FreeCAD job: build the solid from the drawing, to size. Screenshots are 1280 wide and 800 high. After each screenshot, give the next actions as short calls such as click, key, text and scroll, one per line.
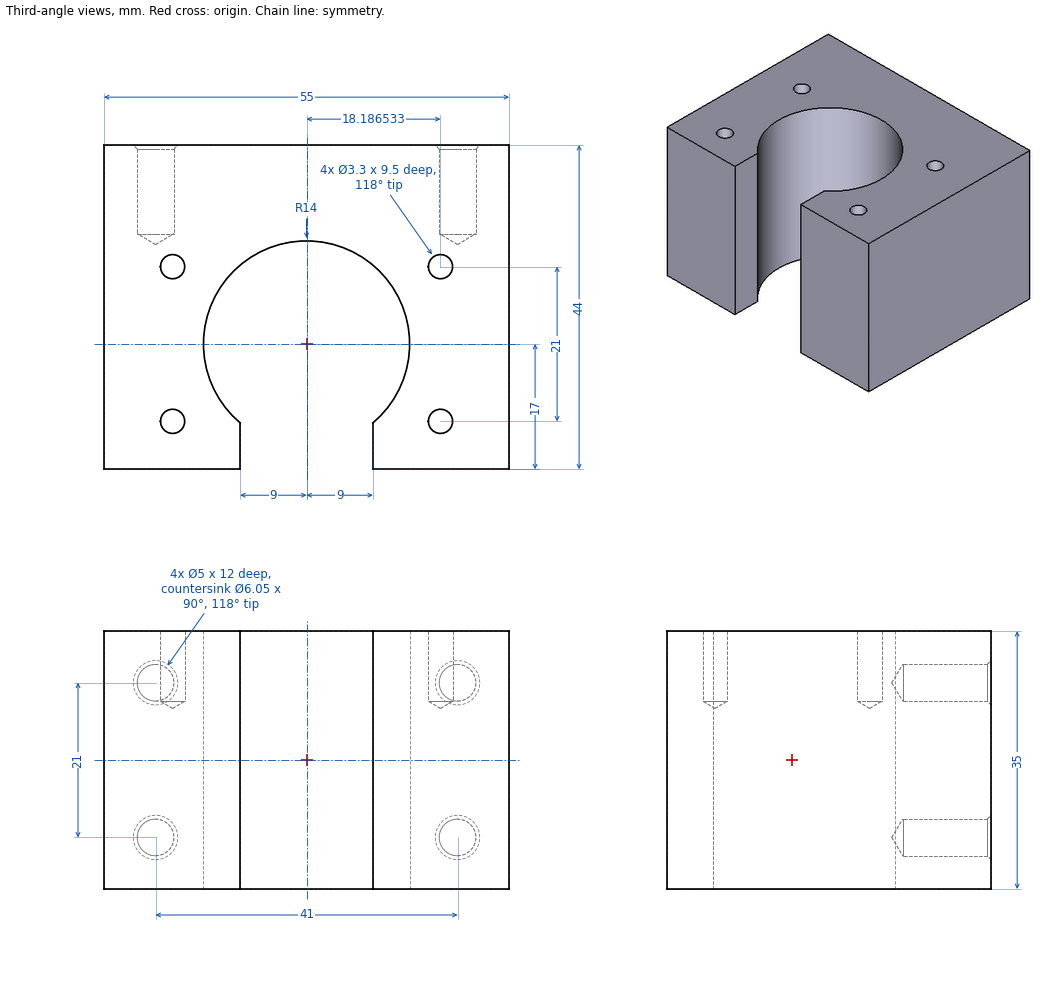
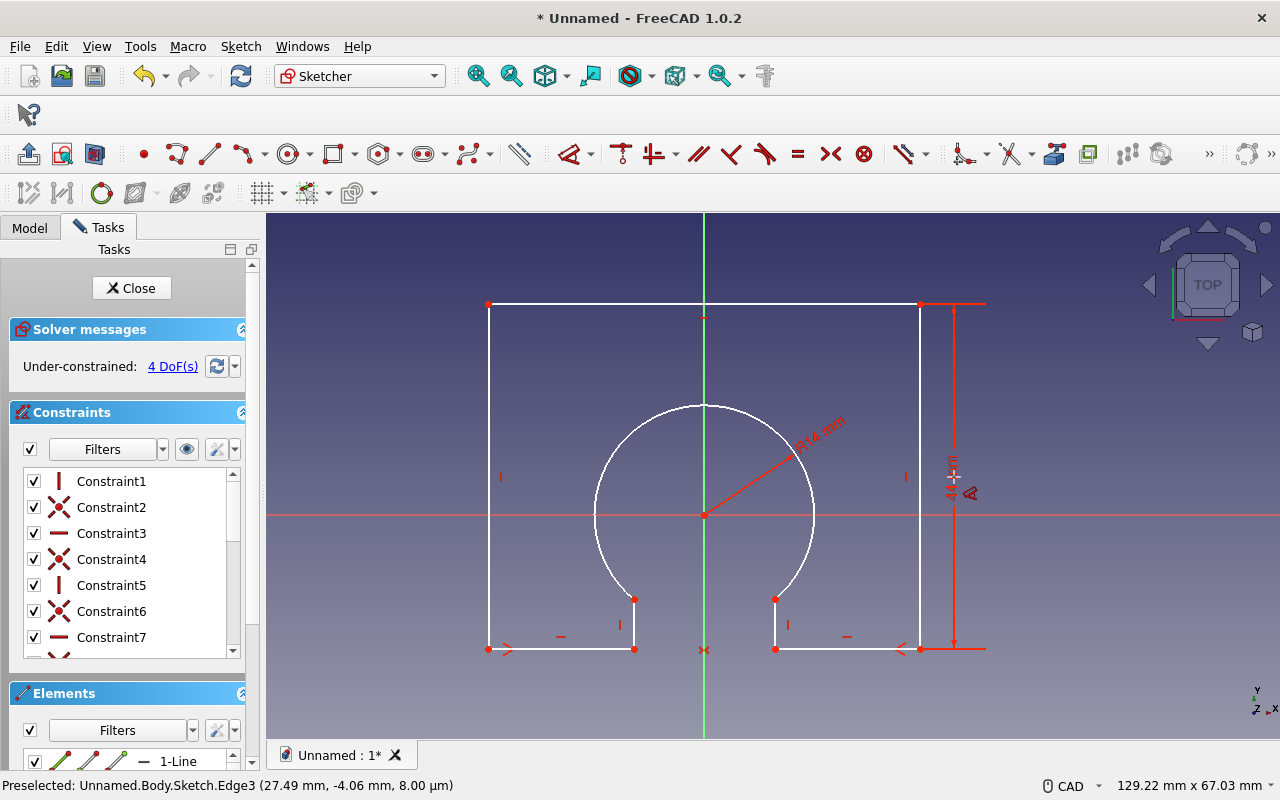
click(791, 304)
click(605, 270)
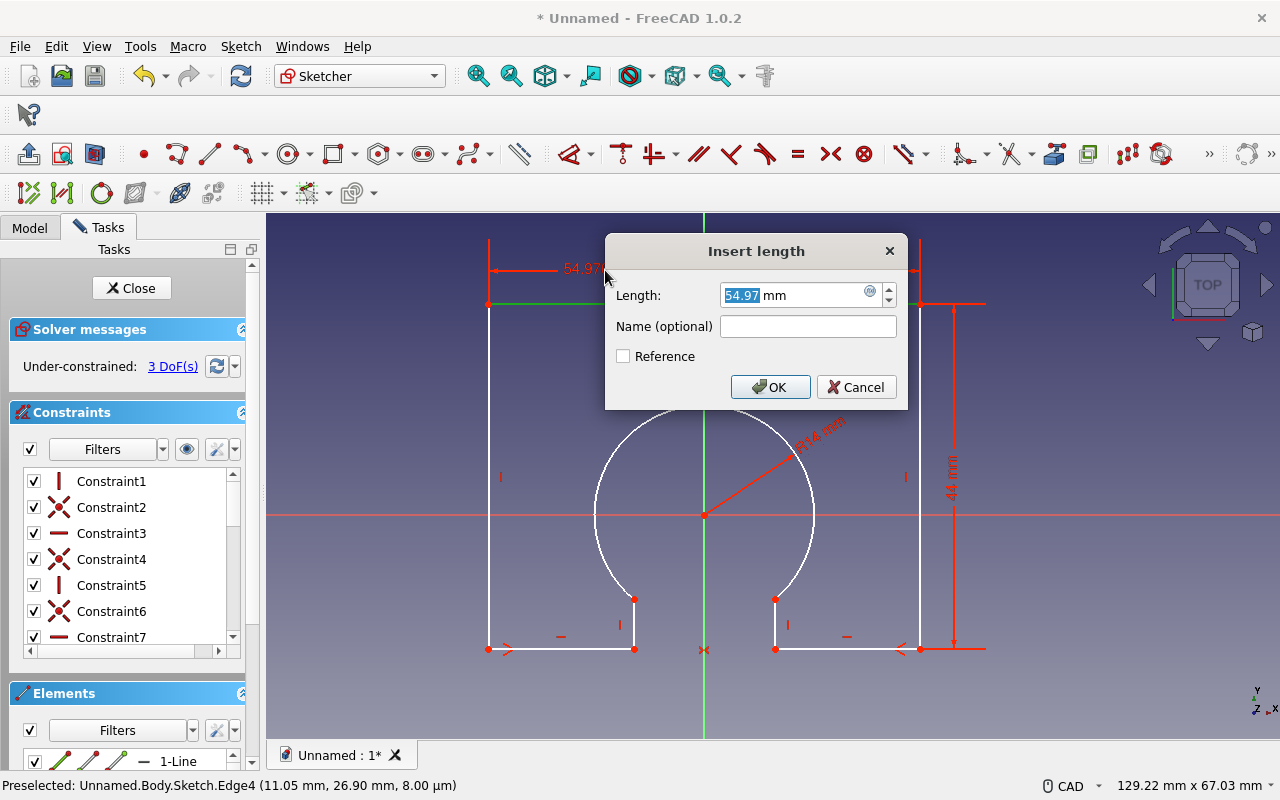
text(55)
key(Return)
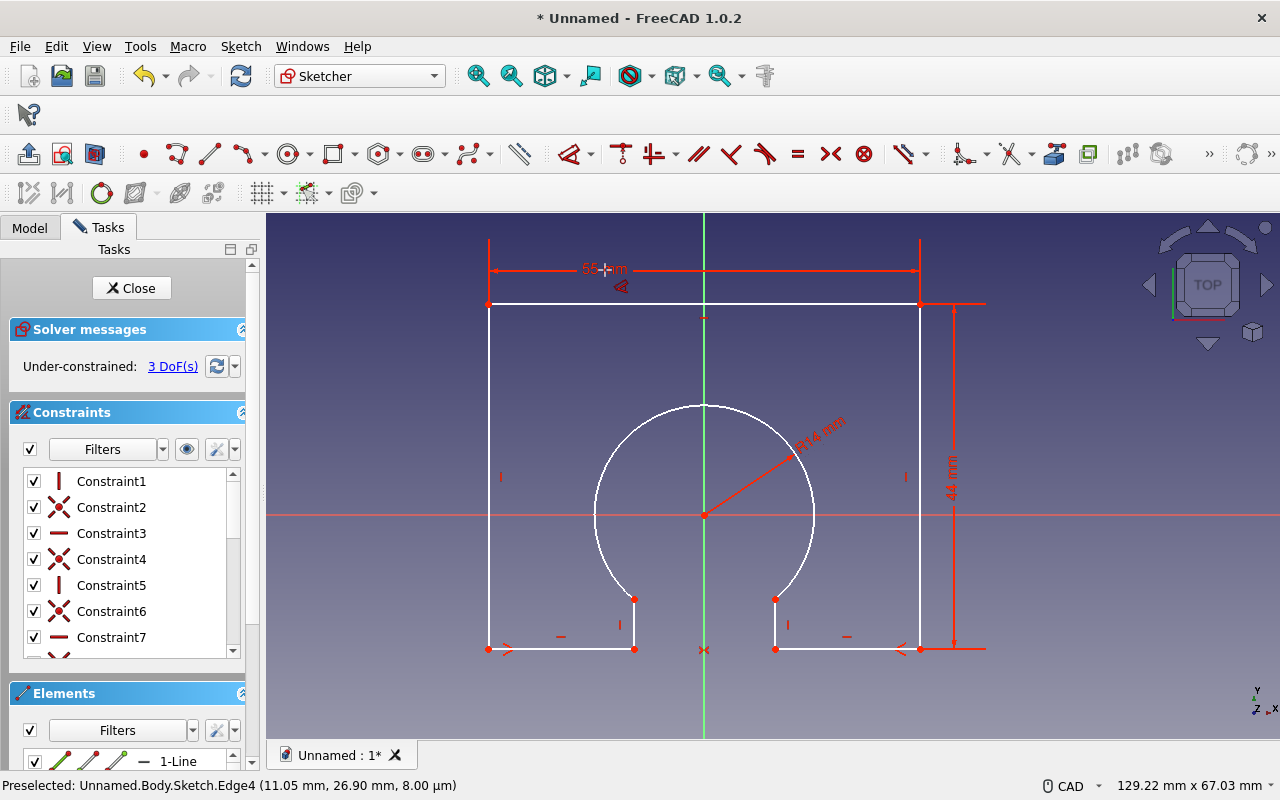
click(775, 599)
click(740, 633)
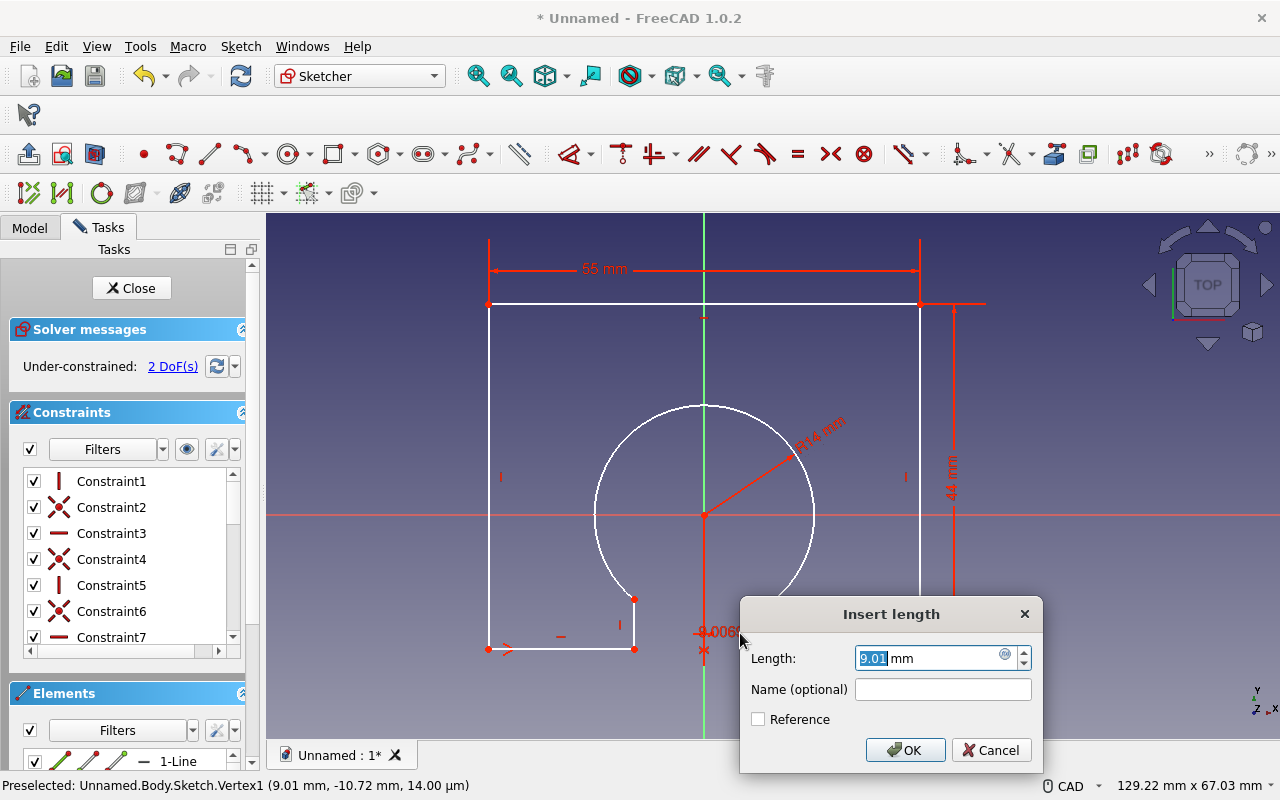
text(9)
key(Return)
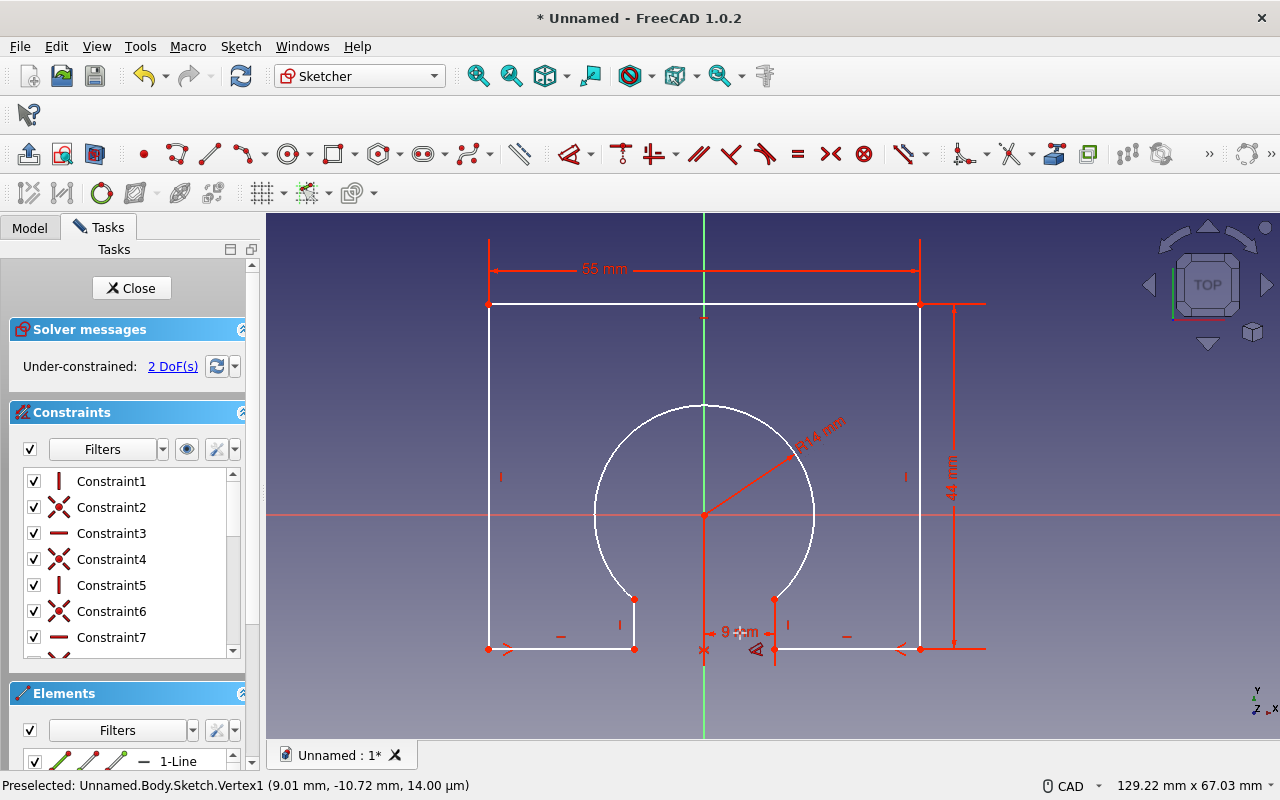
click(634, 649)
click(669, 683)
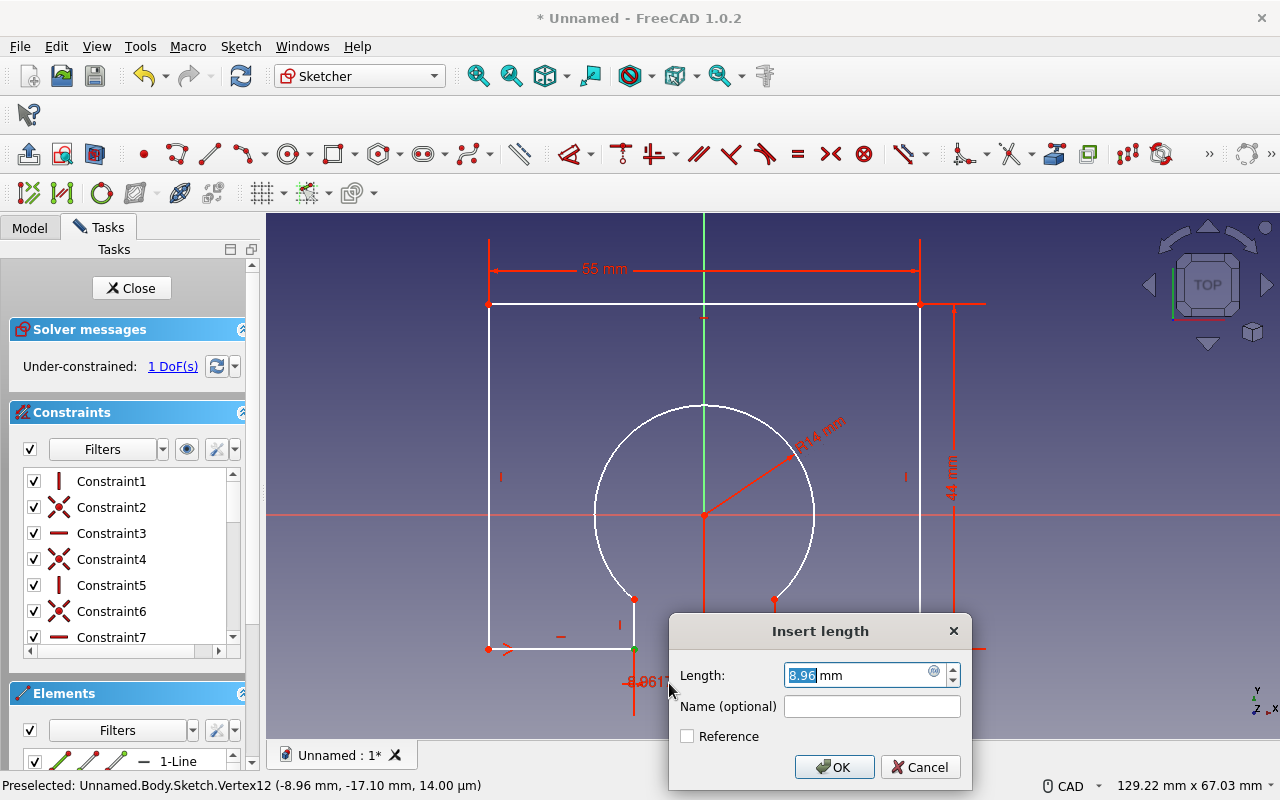
text(9)
key(Return)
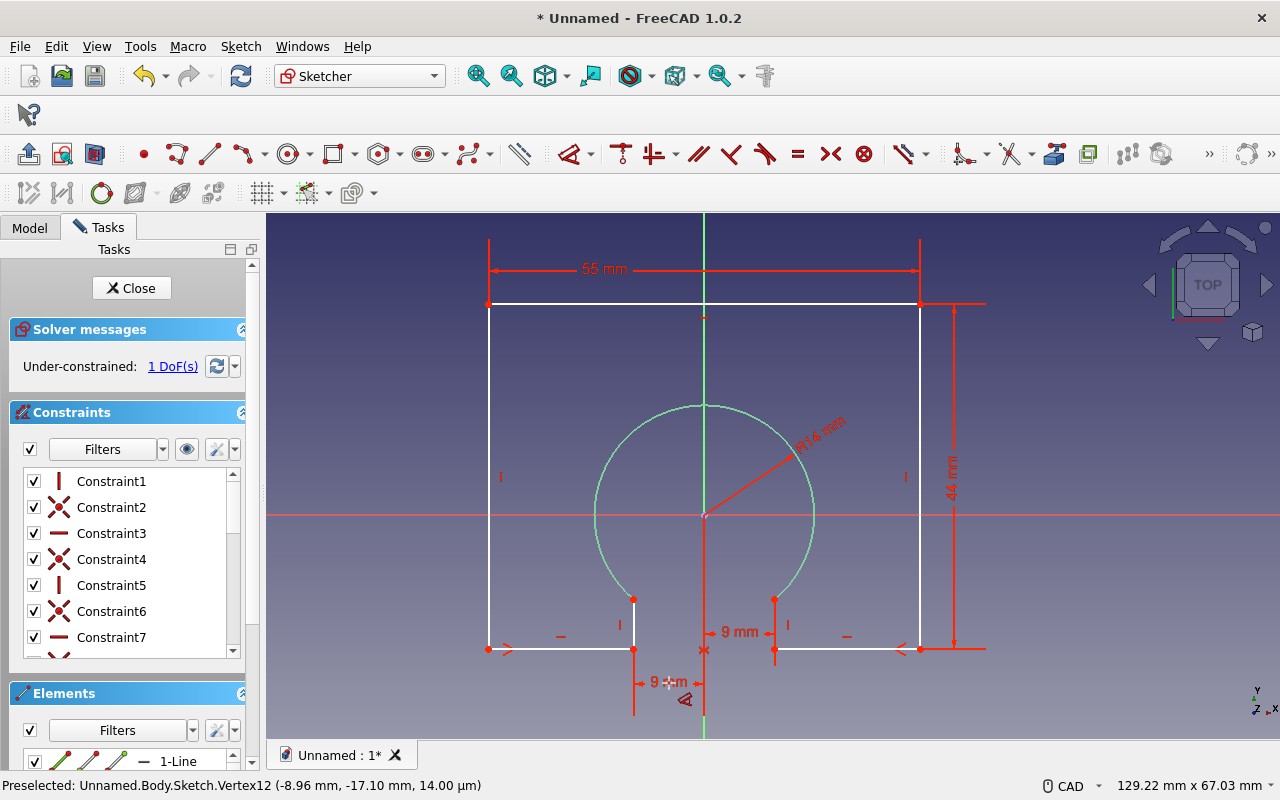
click(775, 649)
click(809, 582)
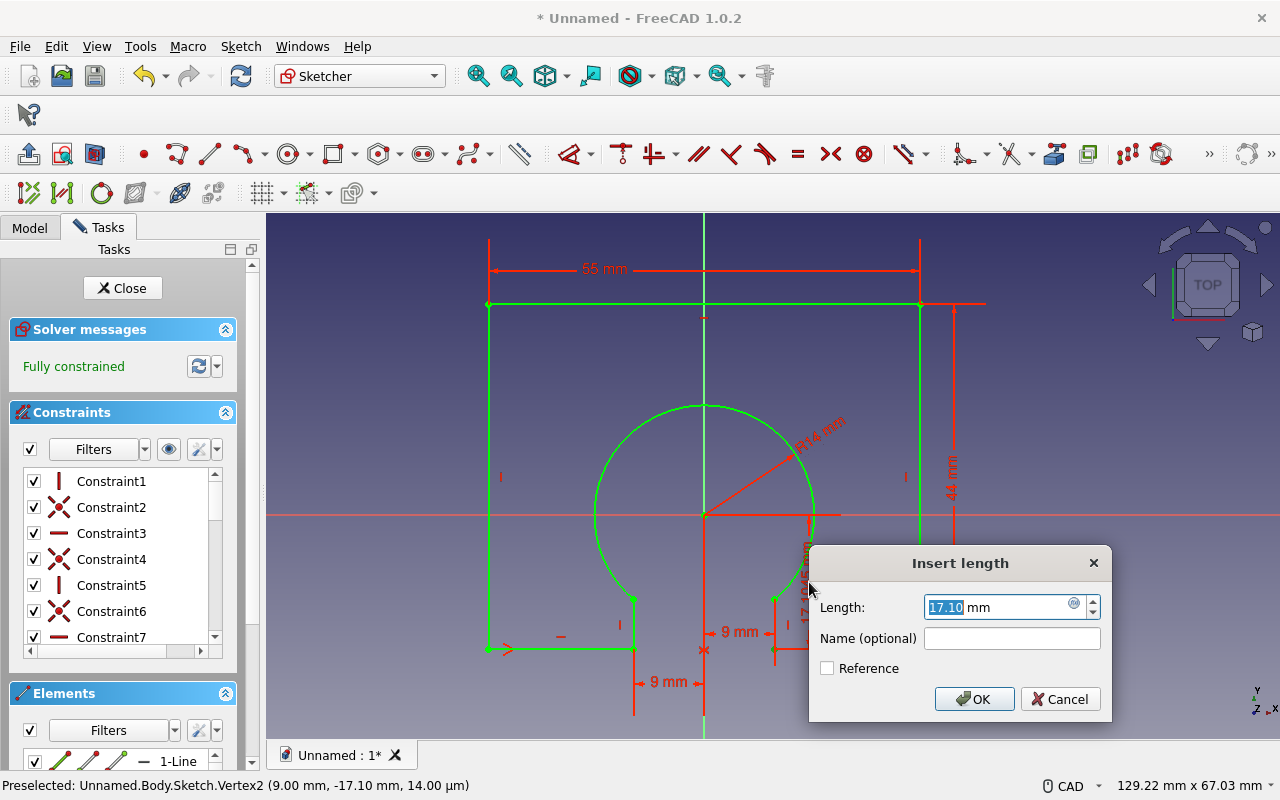
text(17)
key(Return)
key(Escape)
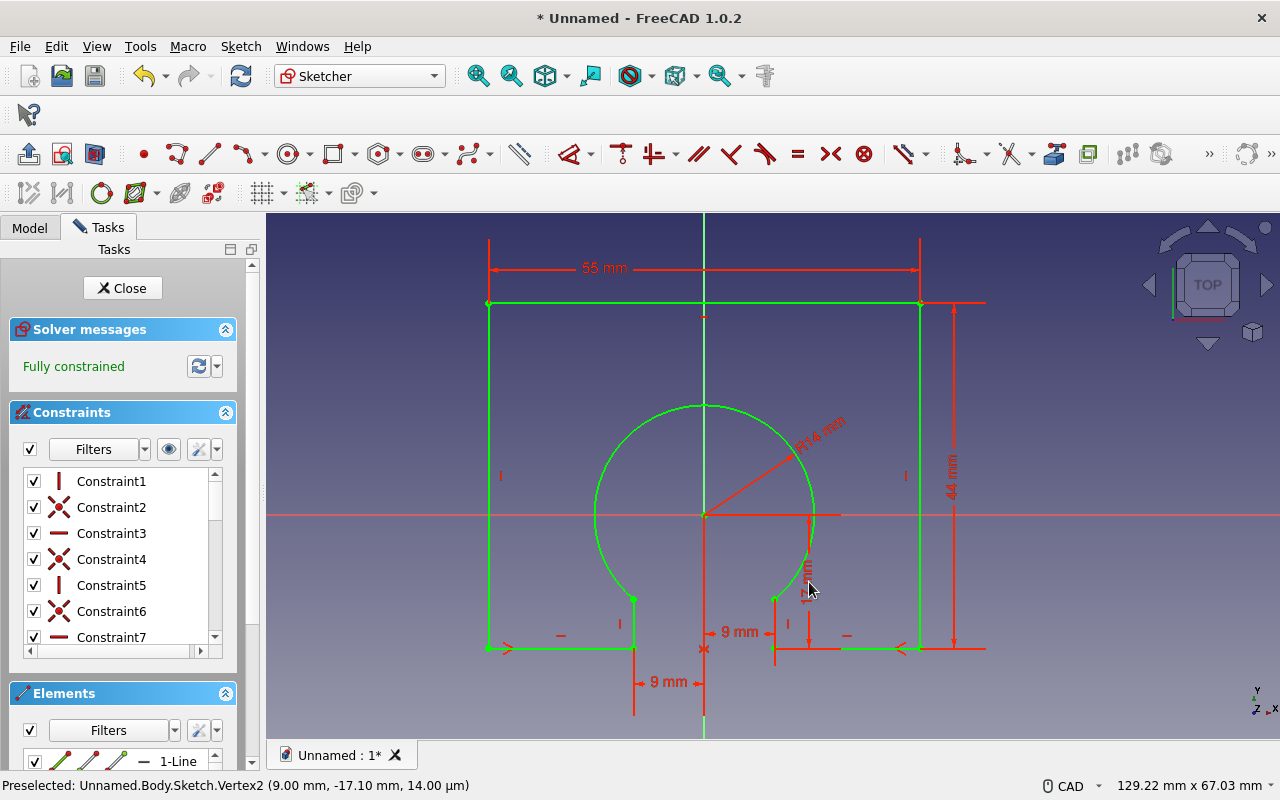
click(123, 288)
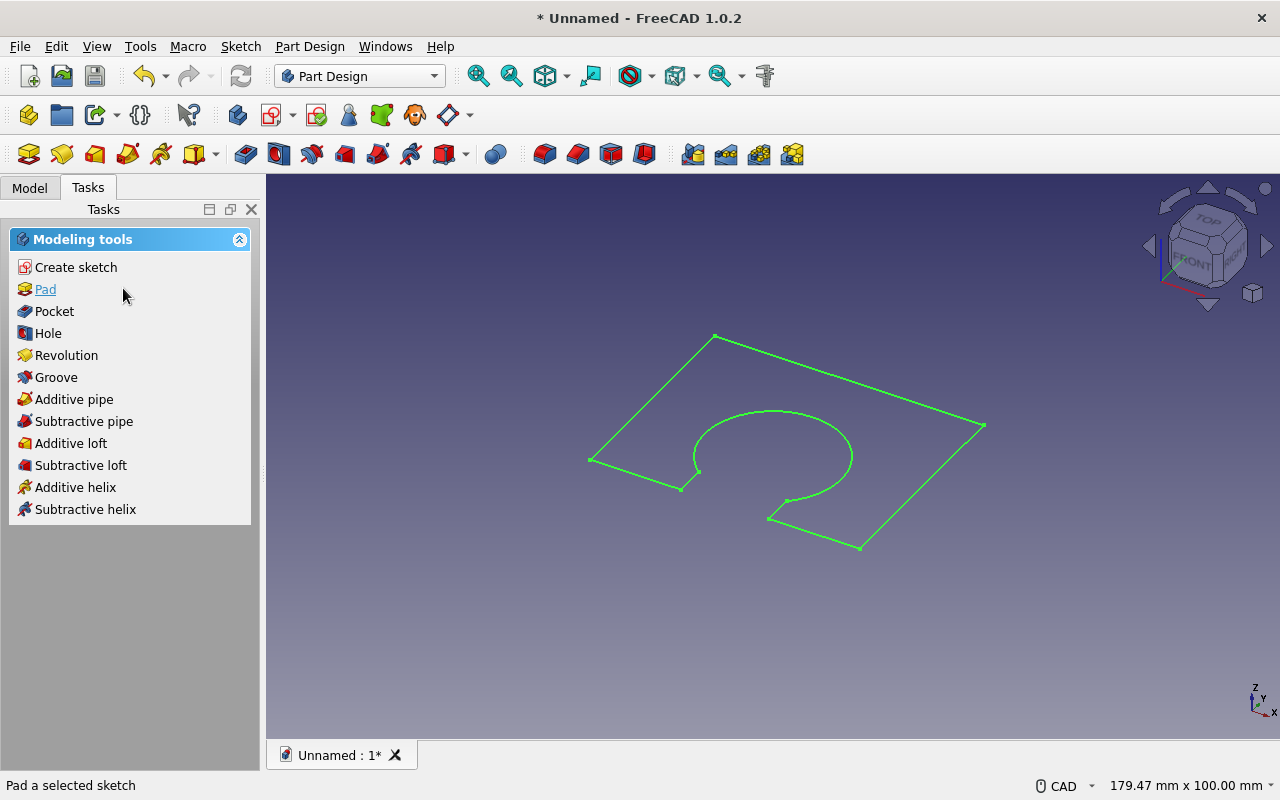
click(29, 154)